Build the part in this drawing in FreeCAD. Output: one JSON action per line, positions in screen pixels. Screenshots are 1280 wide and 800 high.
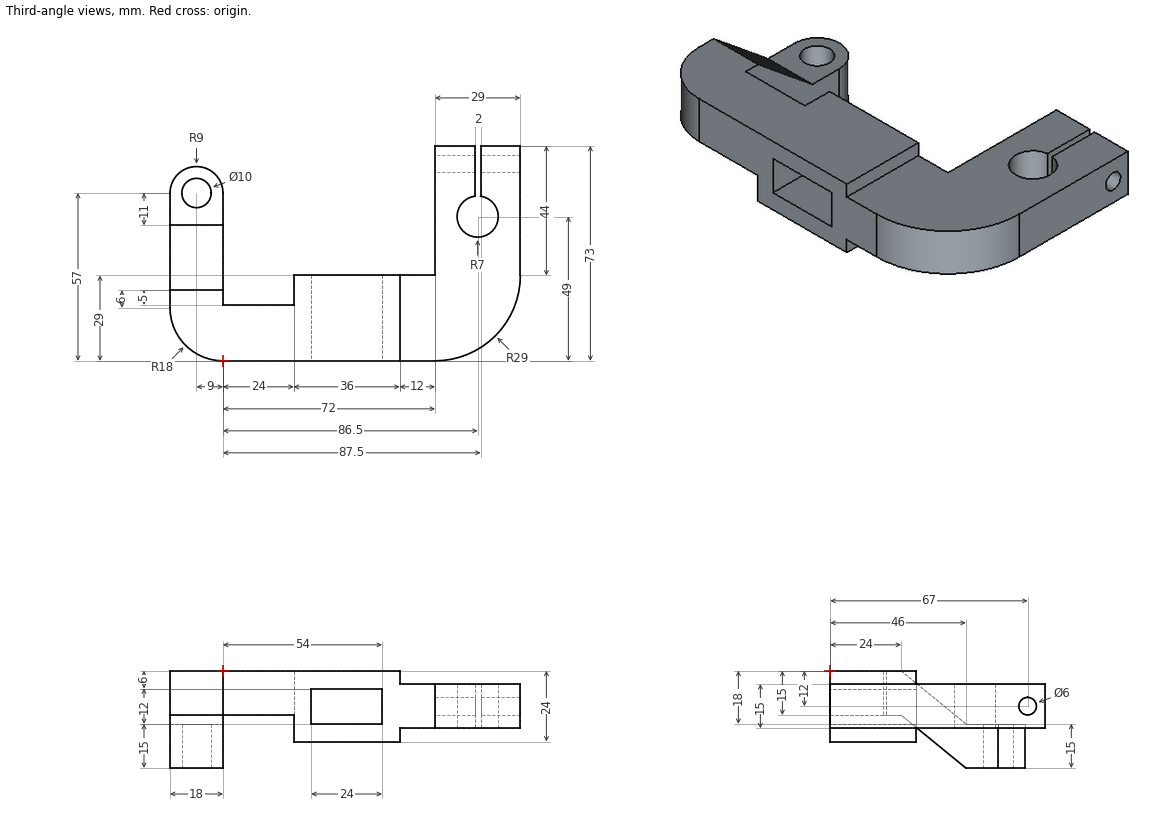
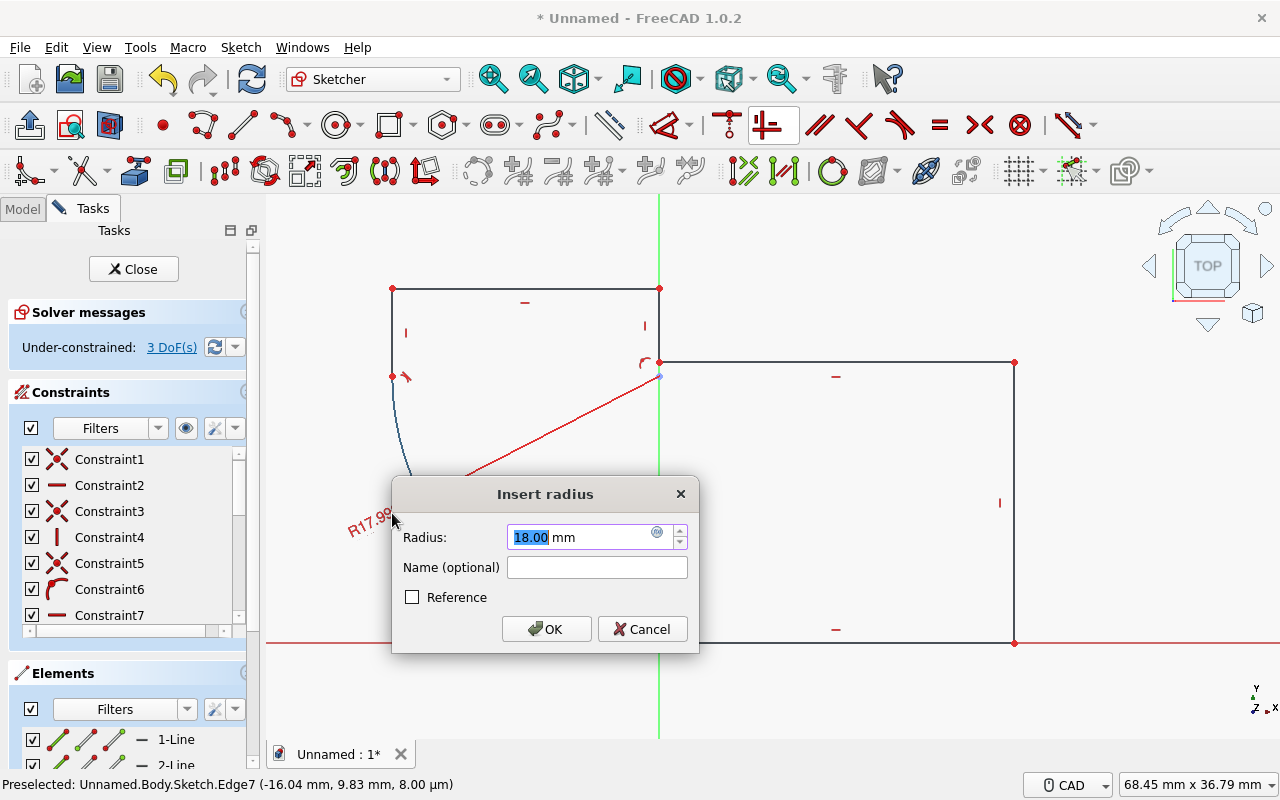
{"action": "type", "text": "18"}
{"action": "key", "text": "Return"}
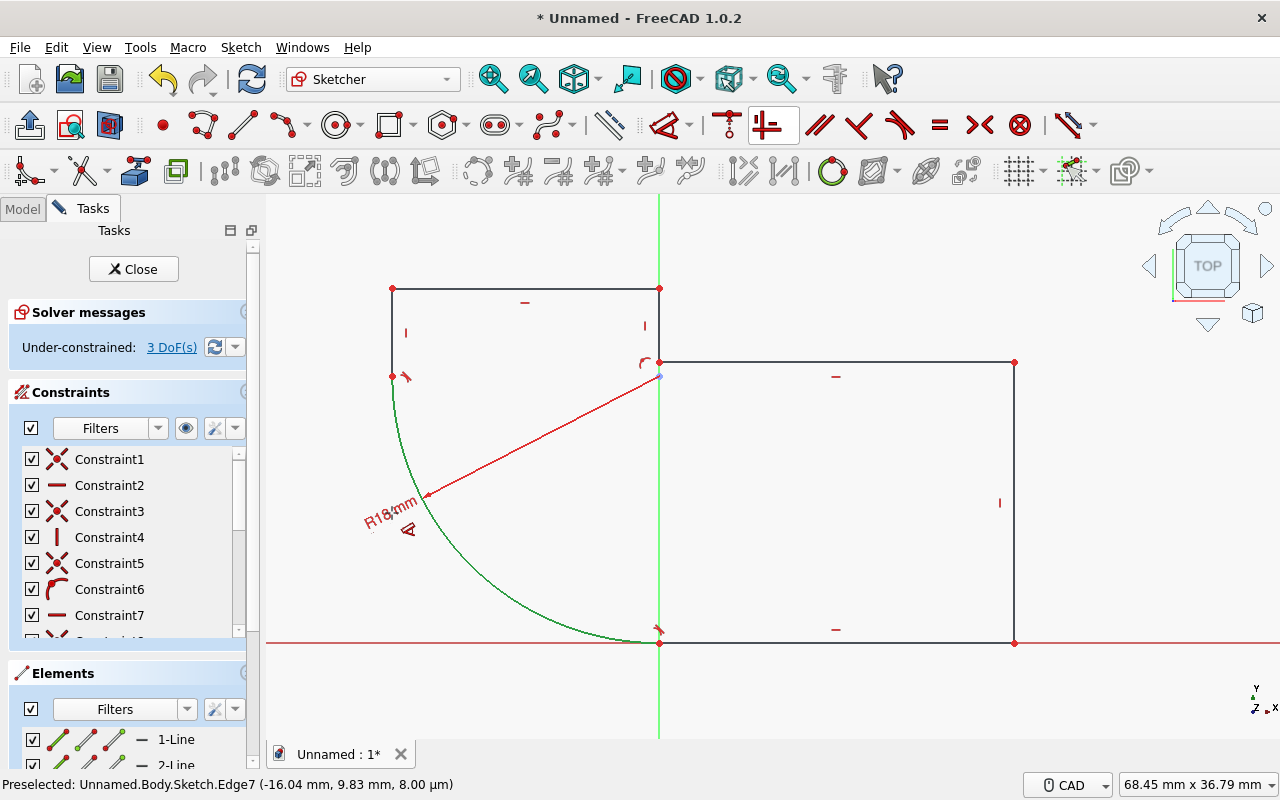
{"action": "left_click", "coordinate": [659, 340]}
{"action": "left_click", "coordinate": [625, 326]}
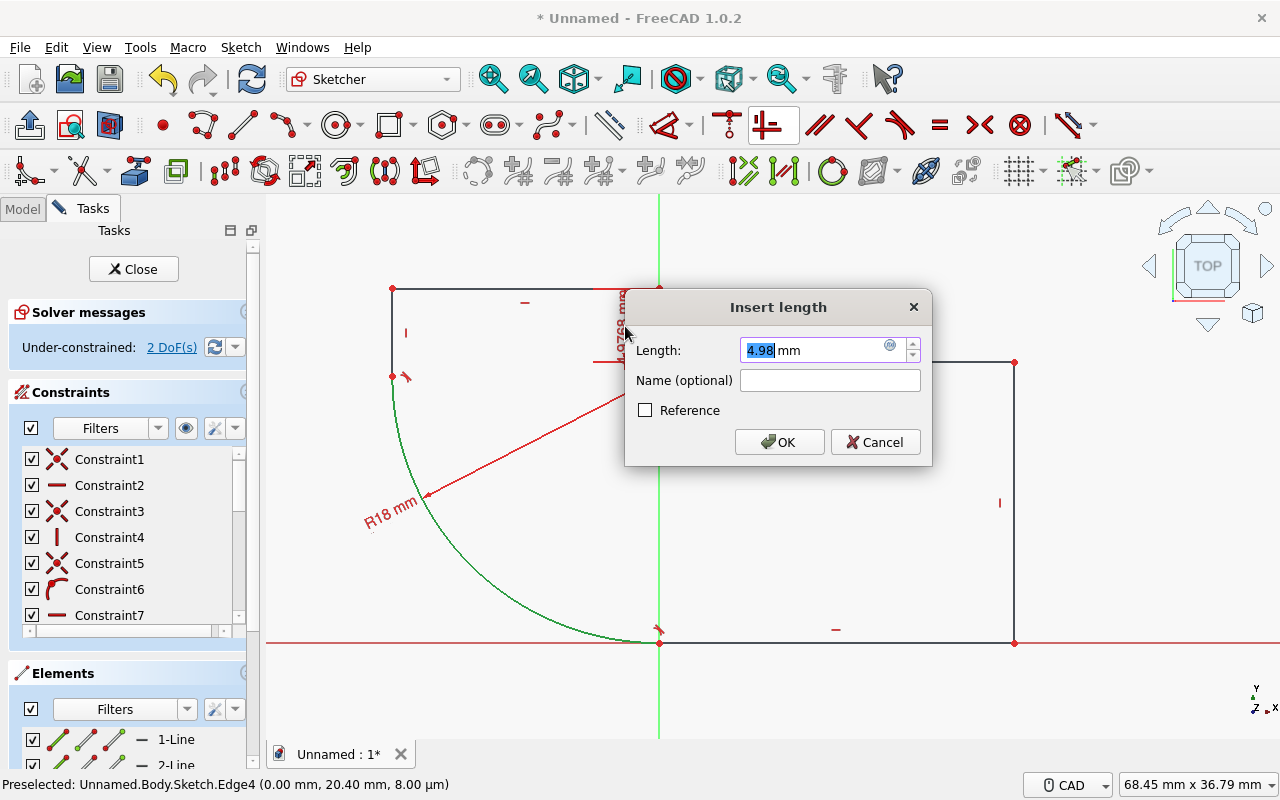
{"action": "type", "text": "5"}
{"action": "key", "text": "Return"}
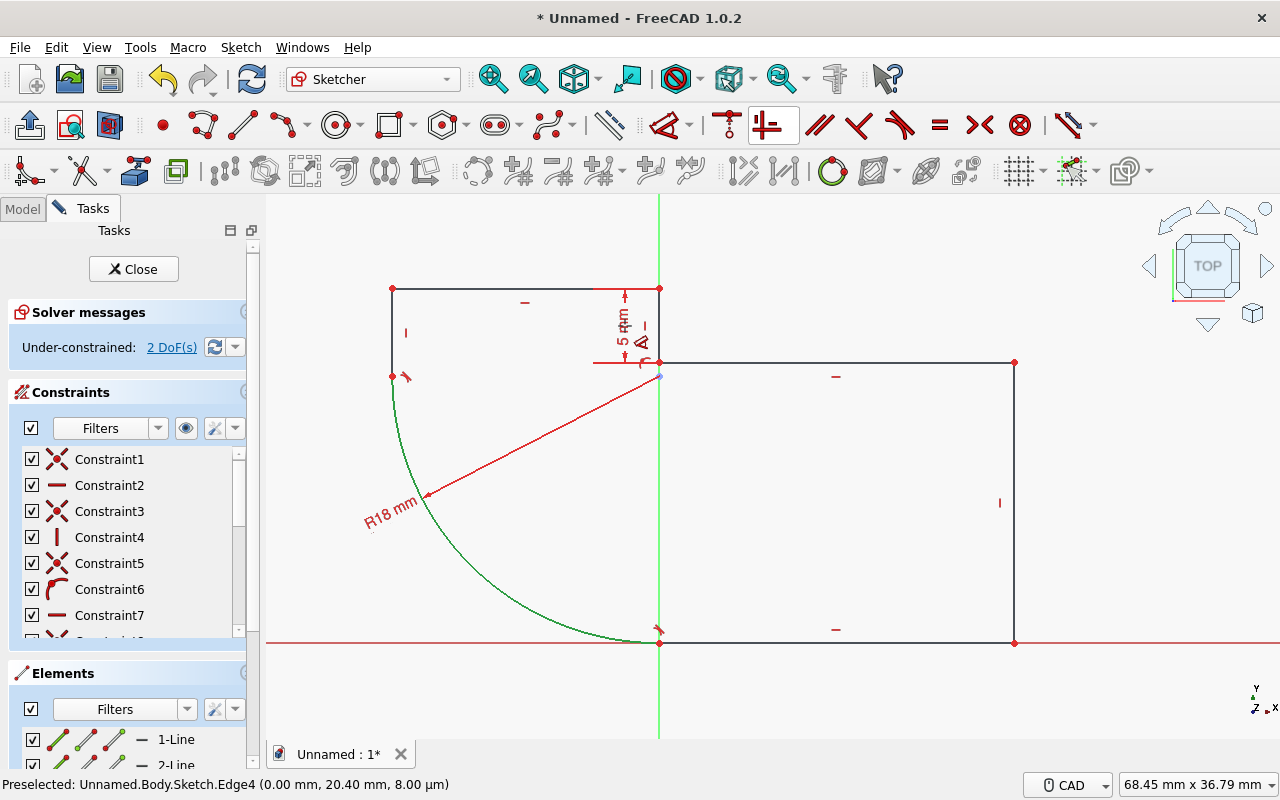
{"action": "left_click", "coordinate": [392, 315]}
{"action": "left_click", "coordinate": [358, 333]}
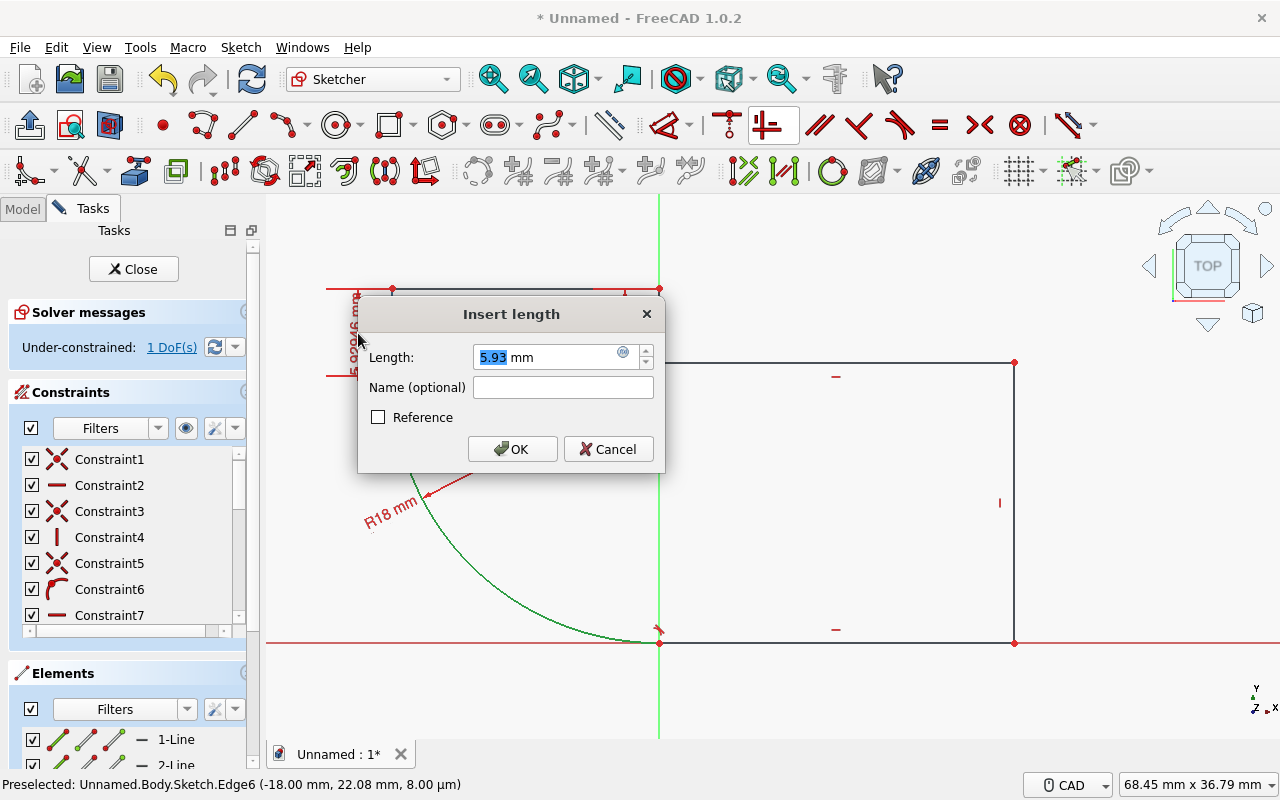
{"action": "type", "text": "6"}
{"action": "key", "text": "Return"}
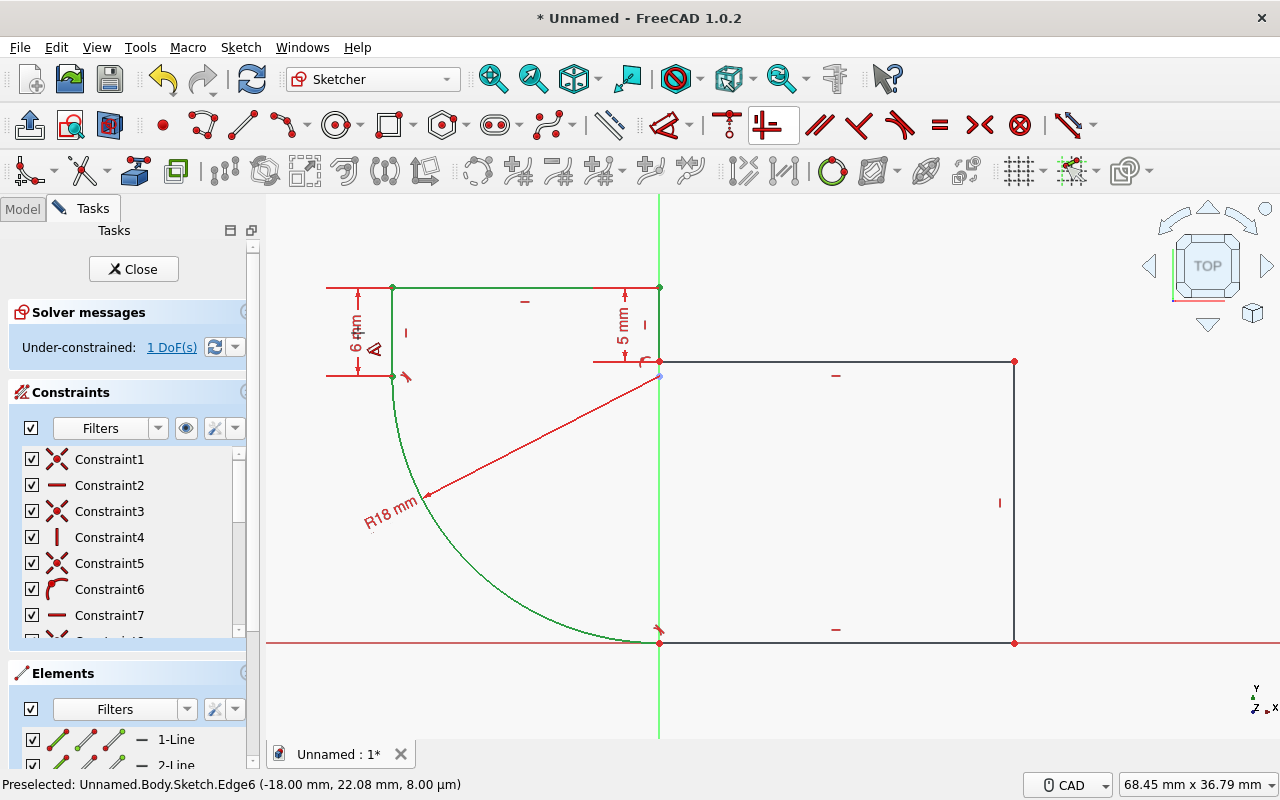
{"action": "left_click", "coordinate": [766, 643]}
{"action": "left_click", "coordinate": [837, 677]}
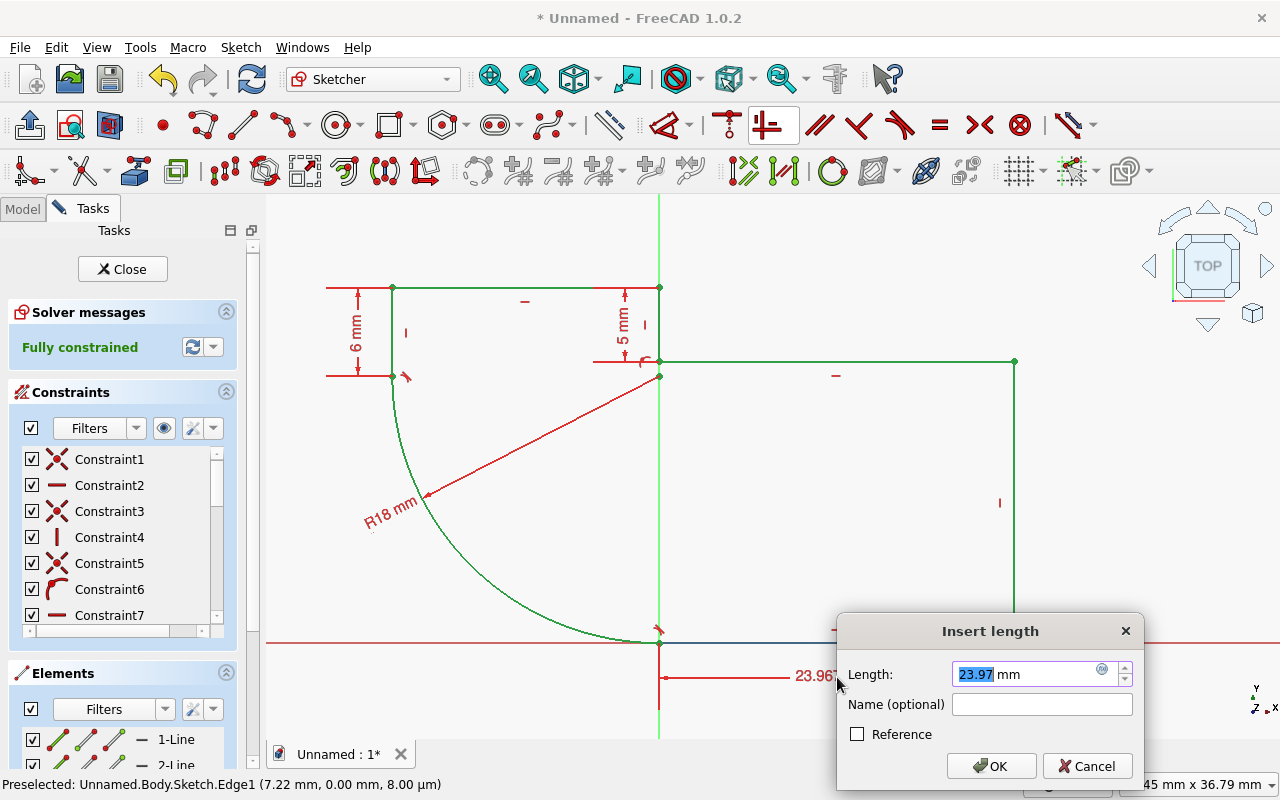
{"action": "type", "text": "24"}
{"action": "key", "text": "Return"}
{"action": "key", "text": "Escape"}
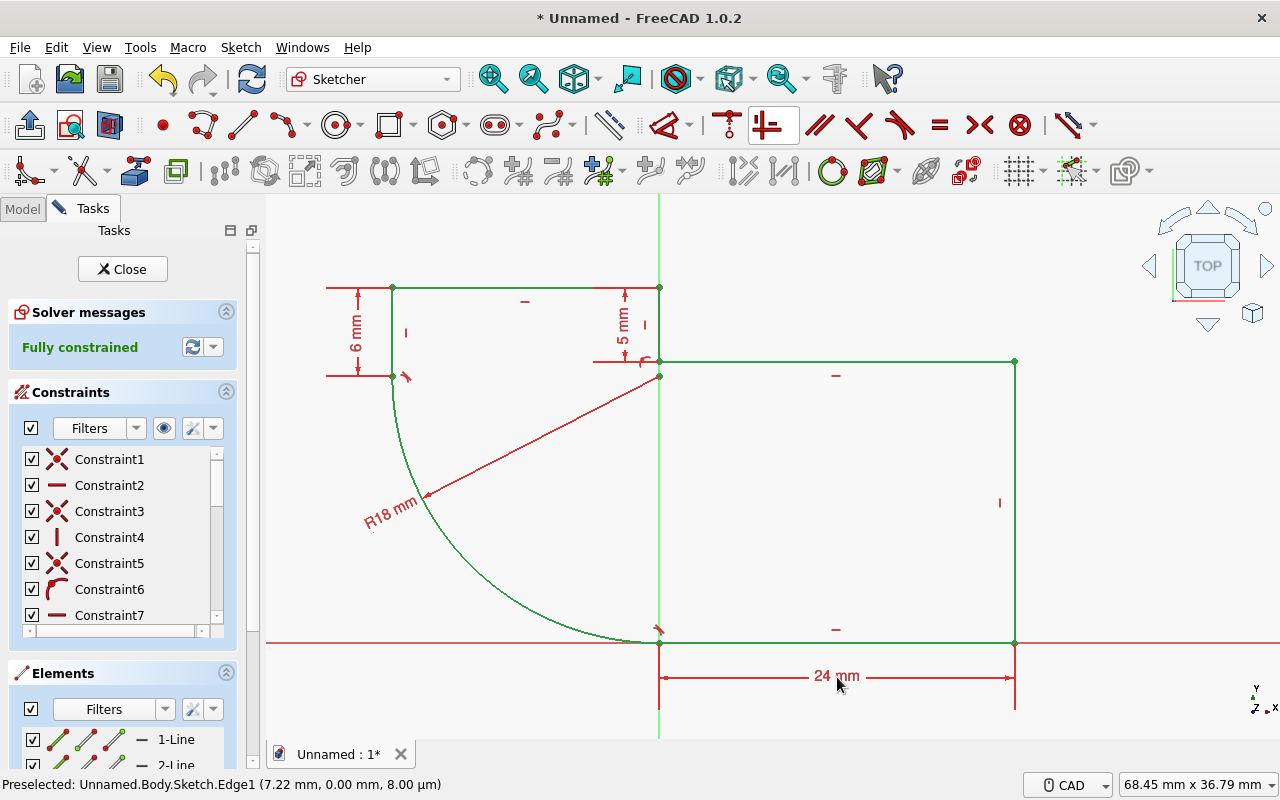
{"action": "left_click", "coordinate": [123, 269]}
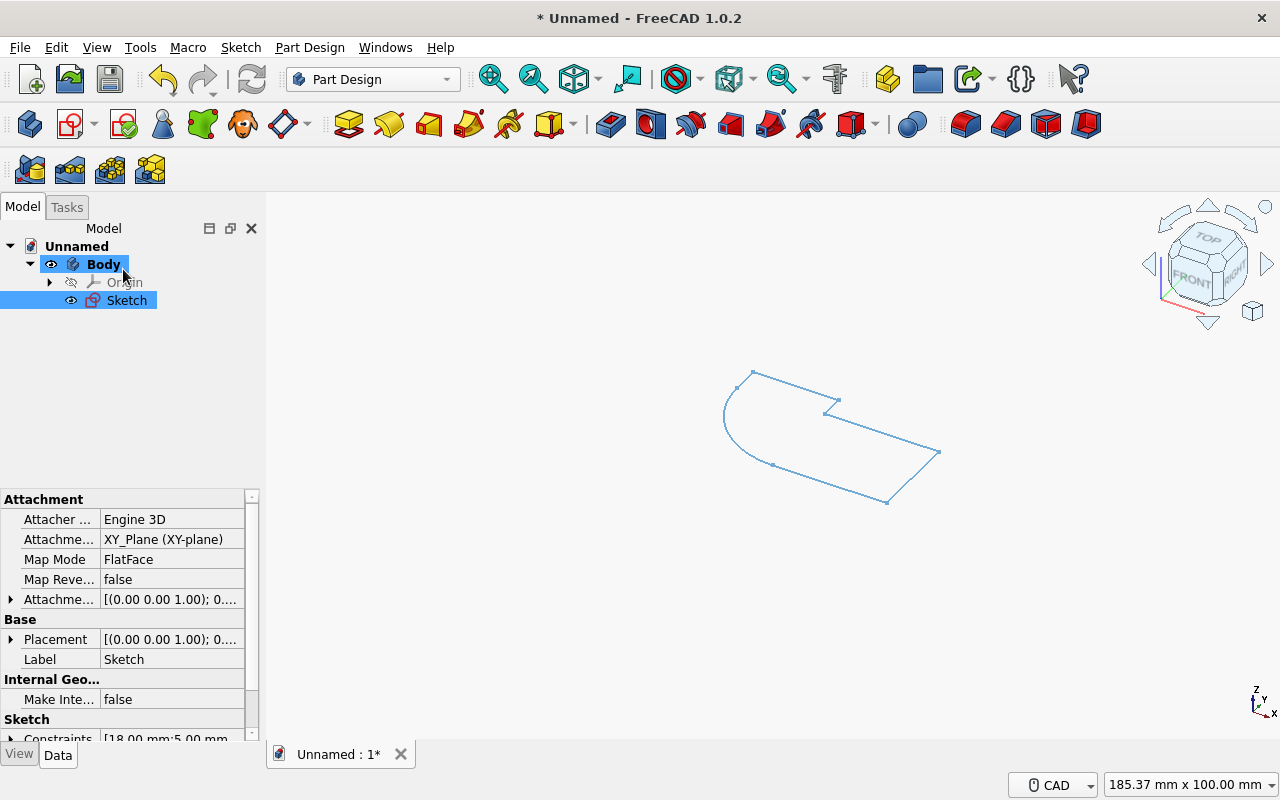
{"action": "left_click", "coordinate": [350, 124]}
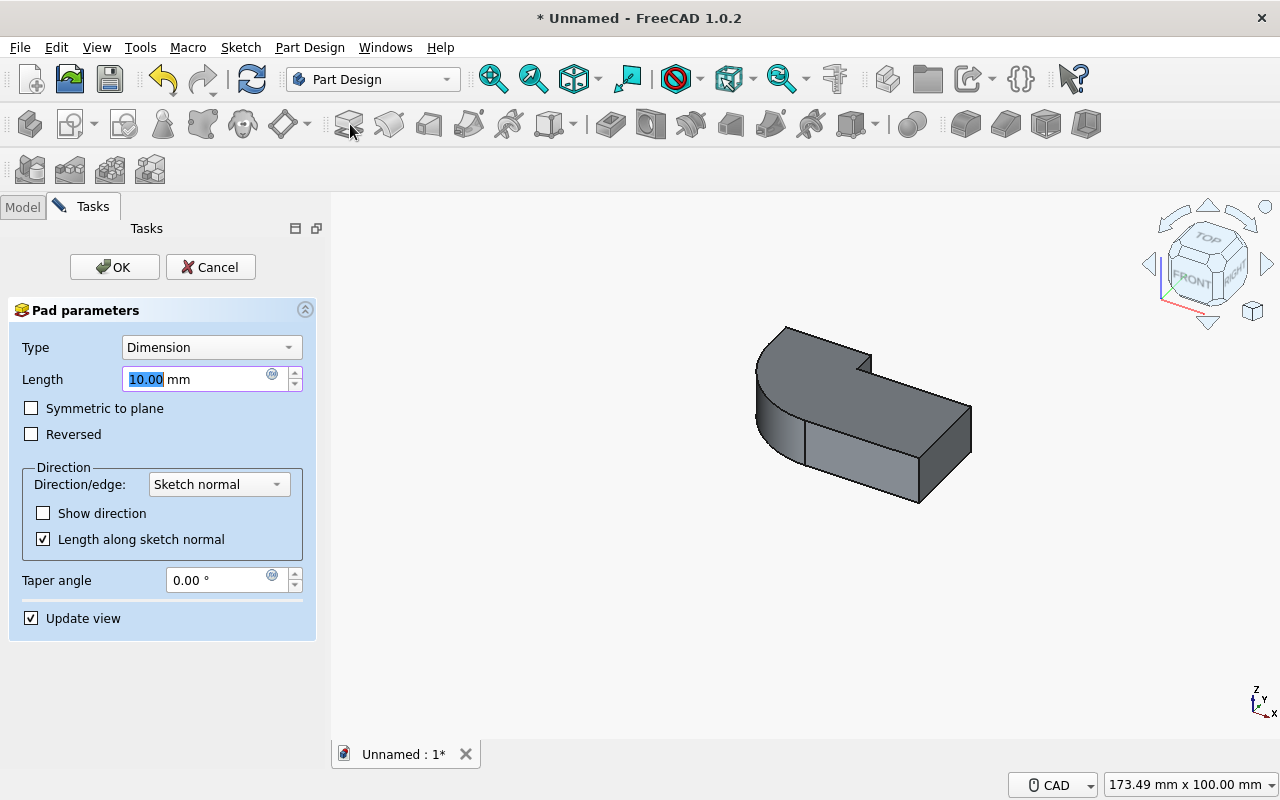
{"action": "type", "text": "15"}
{"action": "key", "text": "Tab"}